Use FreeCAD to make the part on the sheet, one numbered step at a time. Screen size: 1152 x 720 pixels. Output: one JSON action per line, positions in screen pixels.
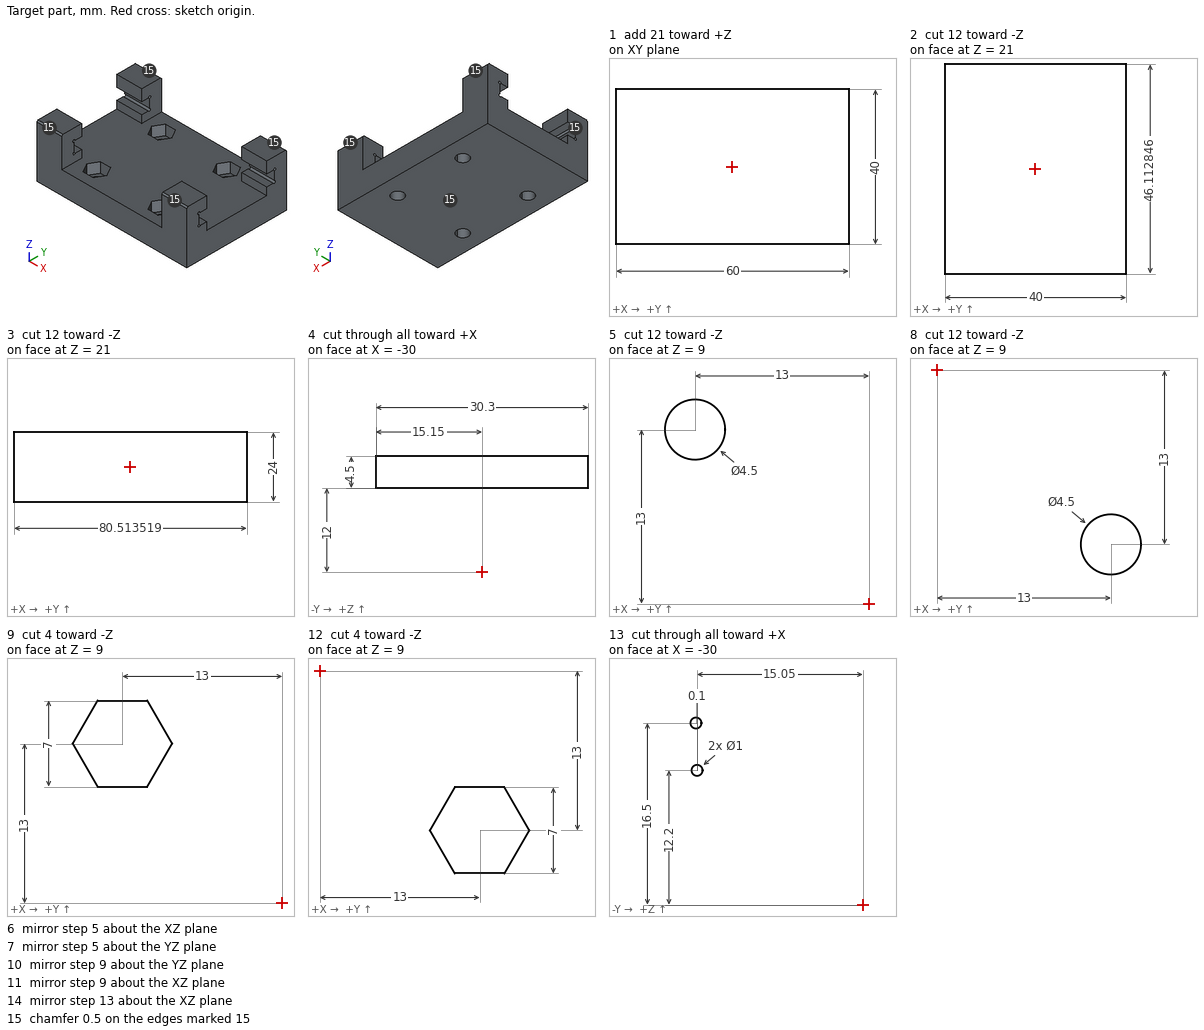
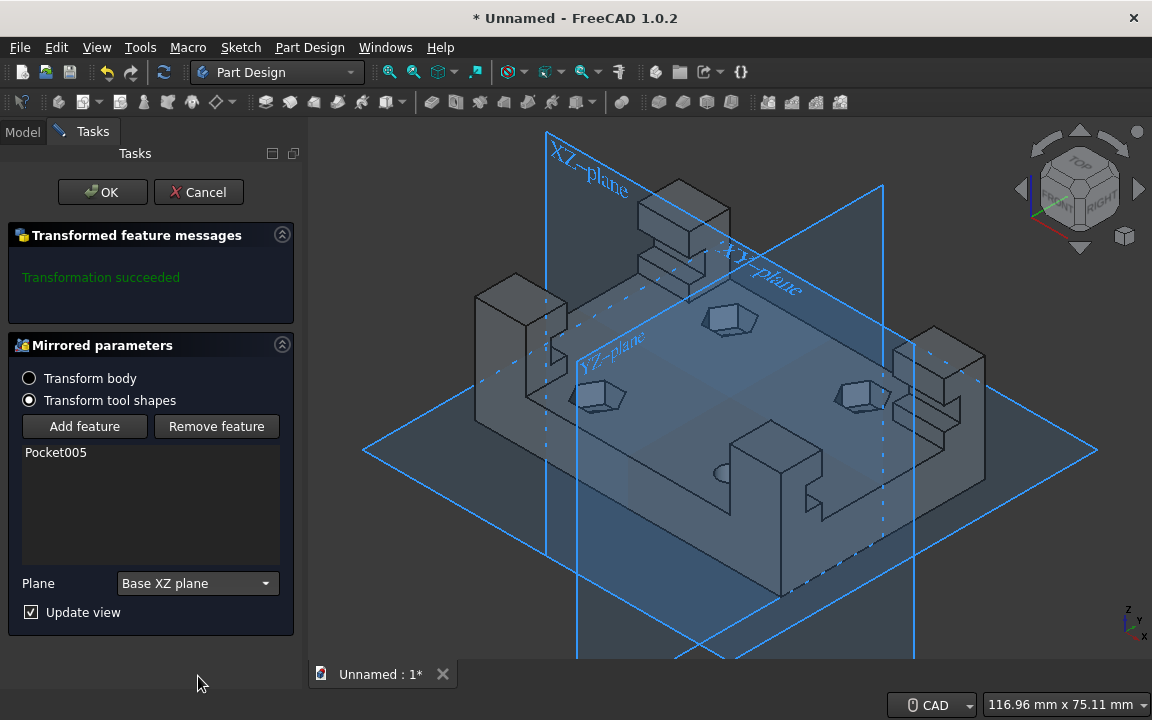
{"action": "left_click", "coordinate": [103, 192]}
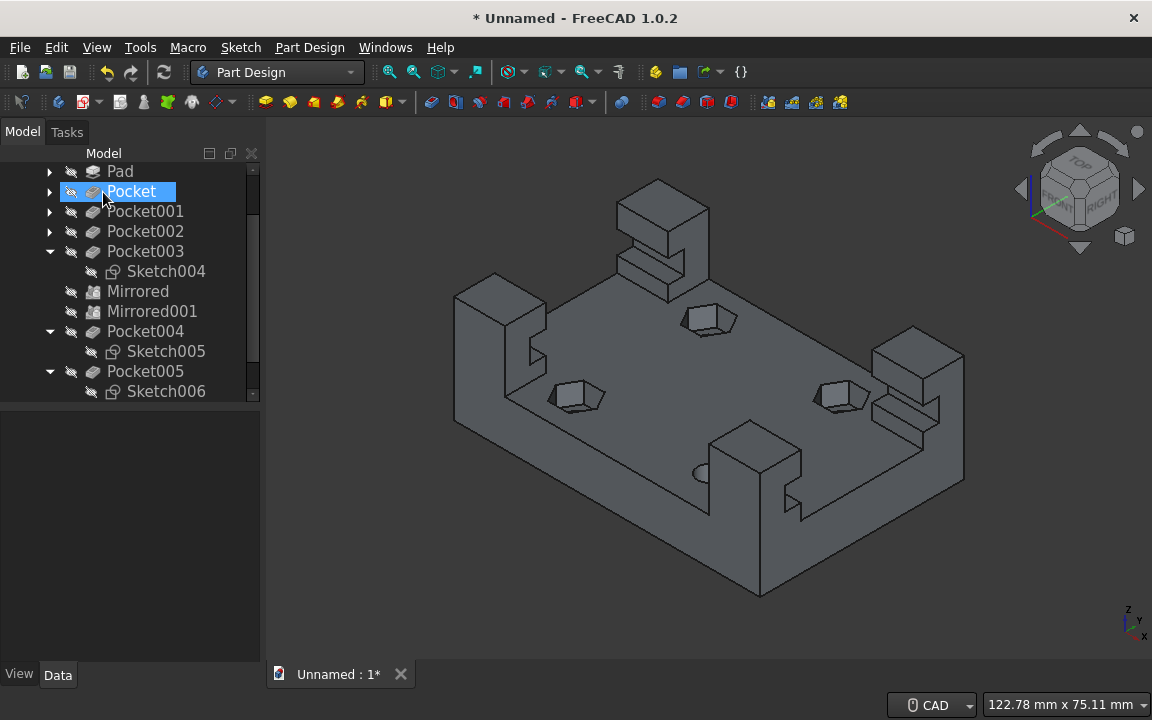
{"action": "left_click", "coordinate": [709, 396]}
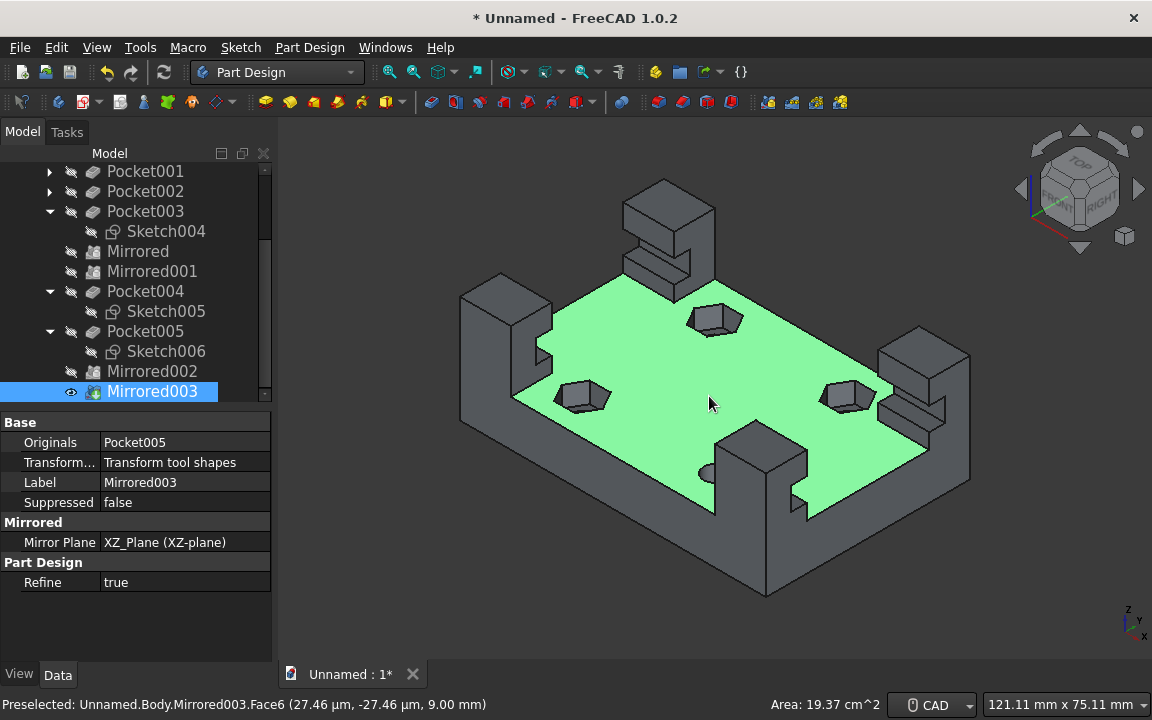
{"action": "left_click", "coordinate": [84, 102]}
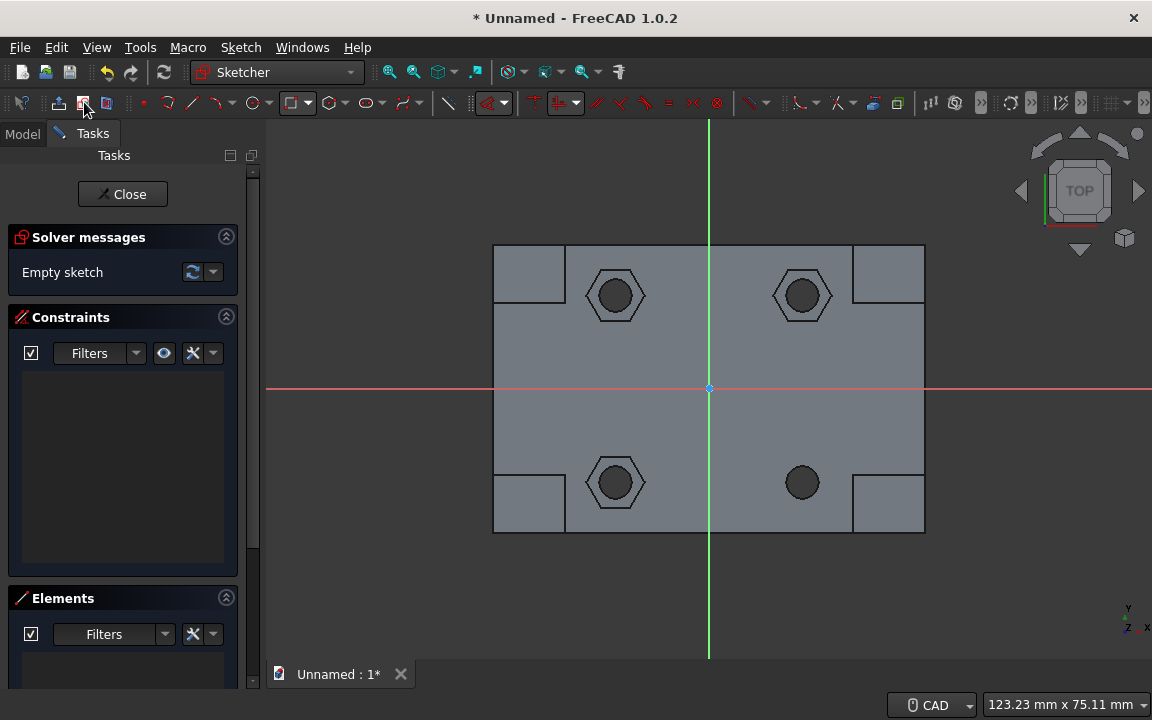
{"action": "left_click", "coordinate": [108, 104]}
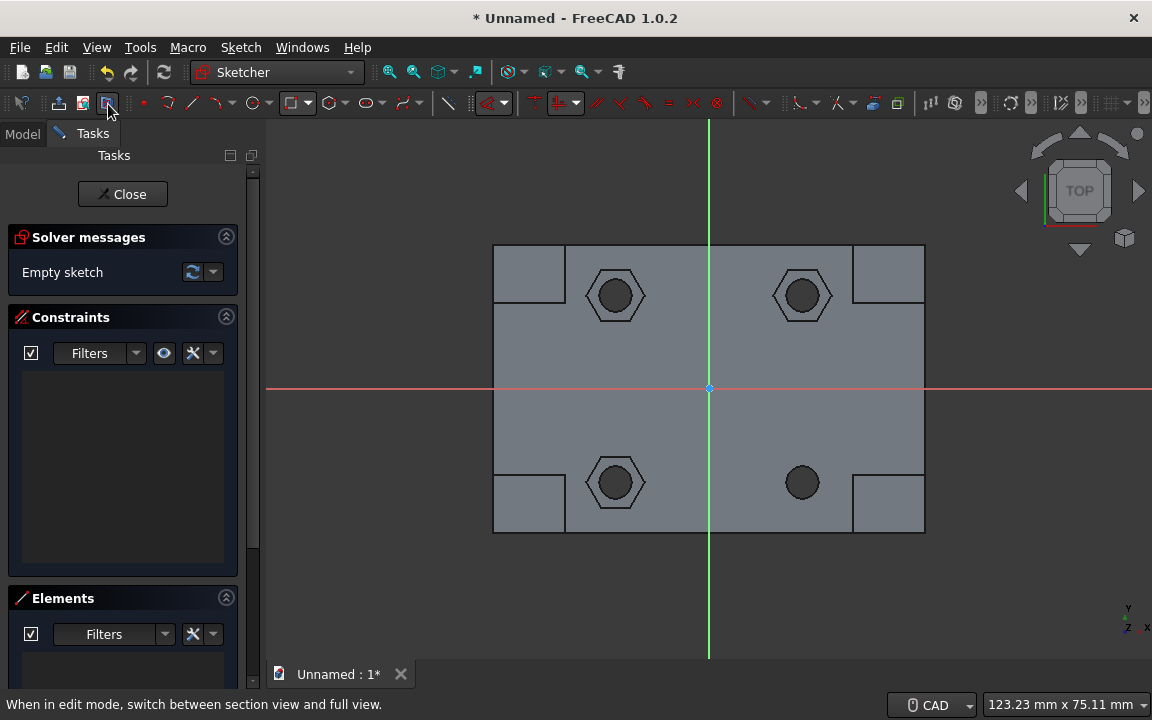
{"action": "scroll", "coordinate": [846, 483], "scroll_direction": "up", "scroll_amount": 5}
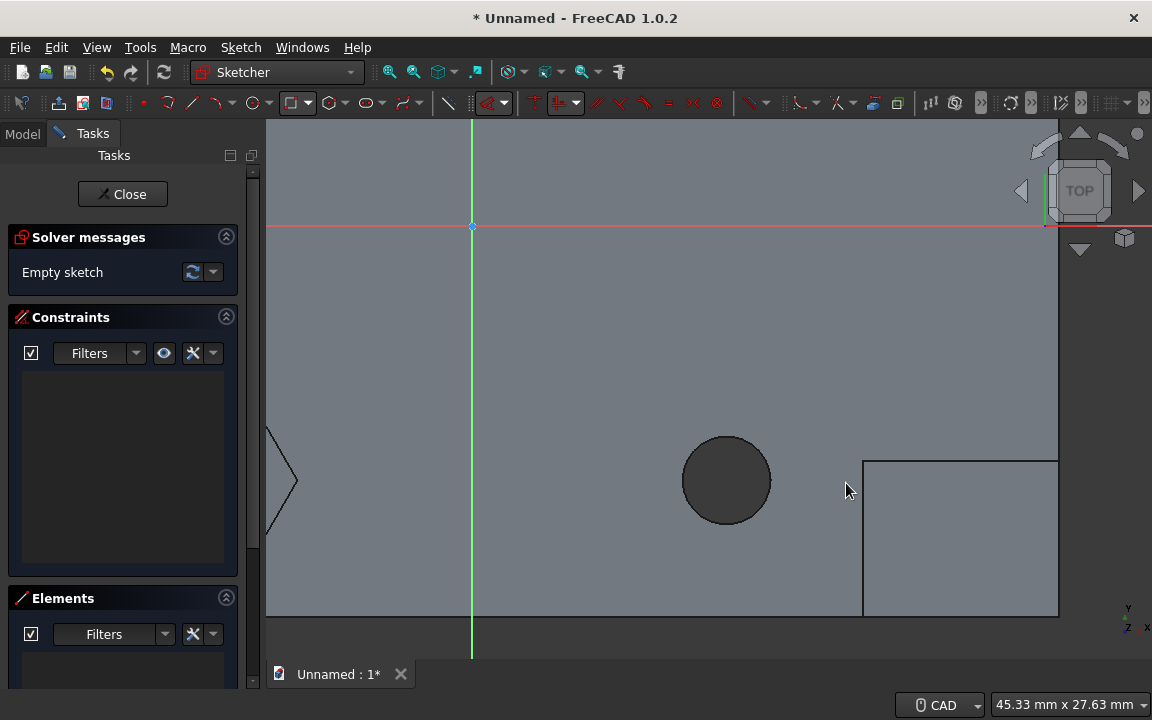
{"action": "left_click", "coordinate": [330, 104]}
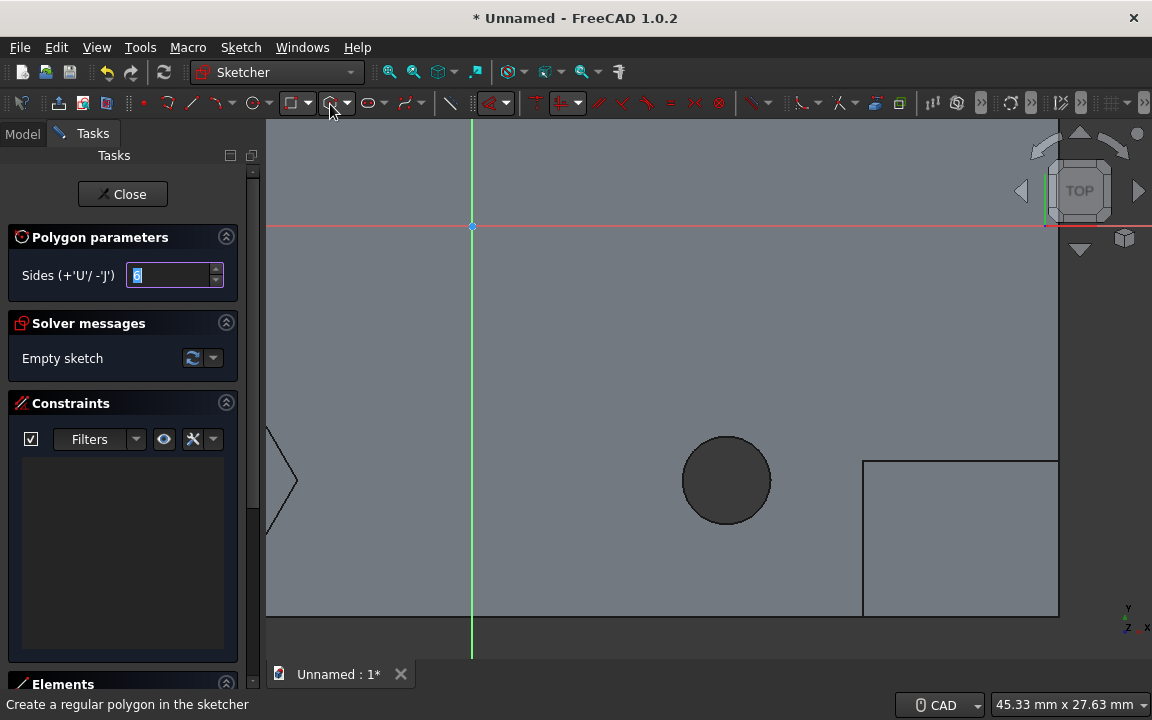
{"action": "left_click", "coordinate": [727, 480]}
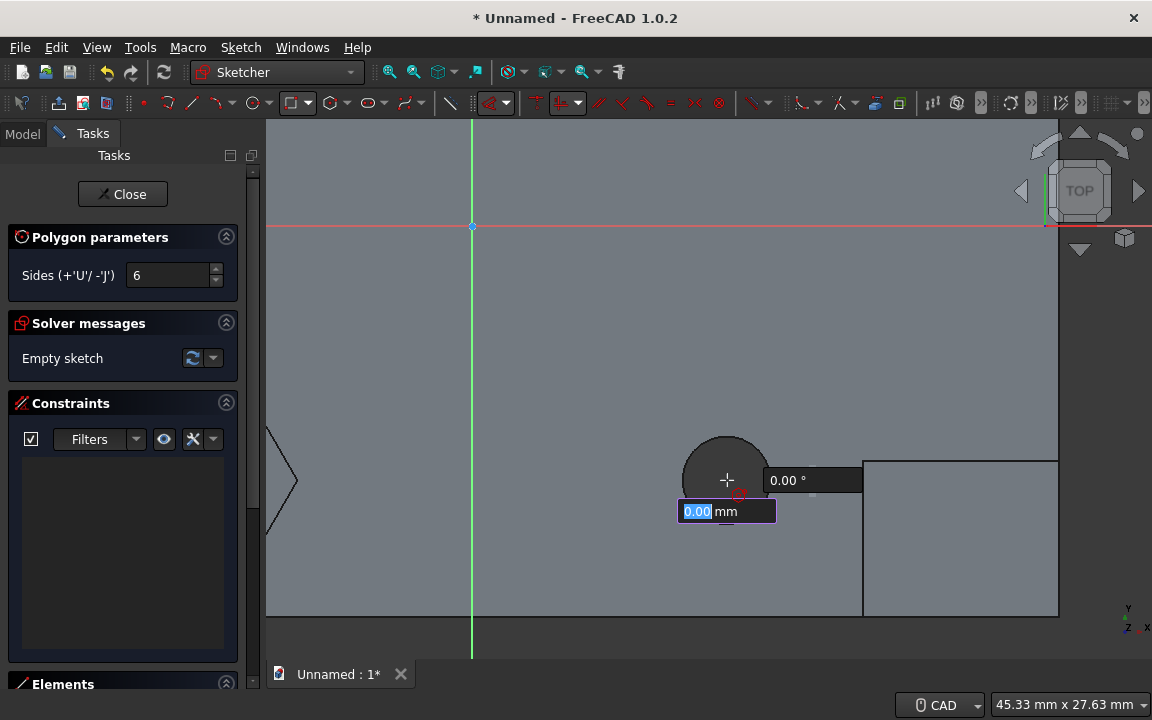
{"action": "left_click", "coordinate": [806, 480]}
{"action": "key", "text": "Escape"}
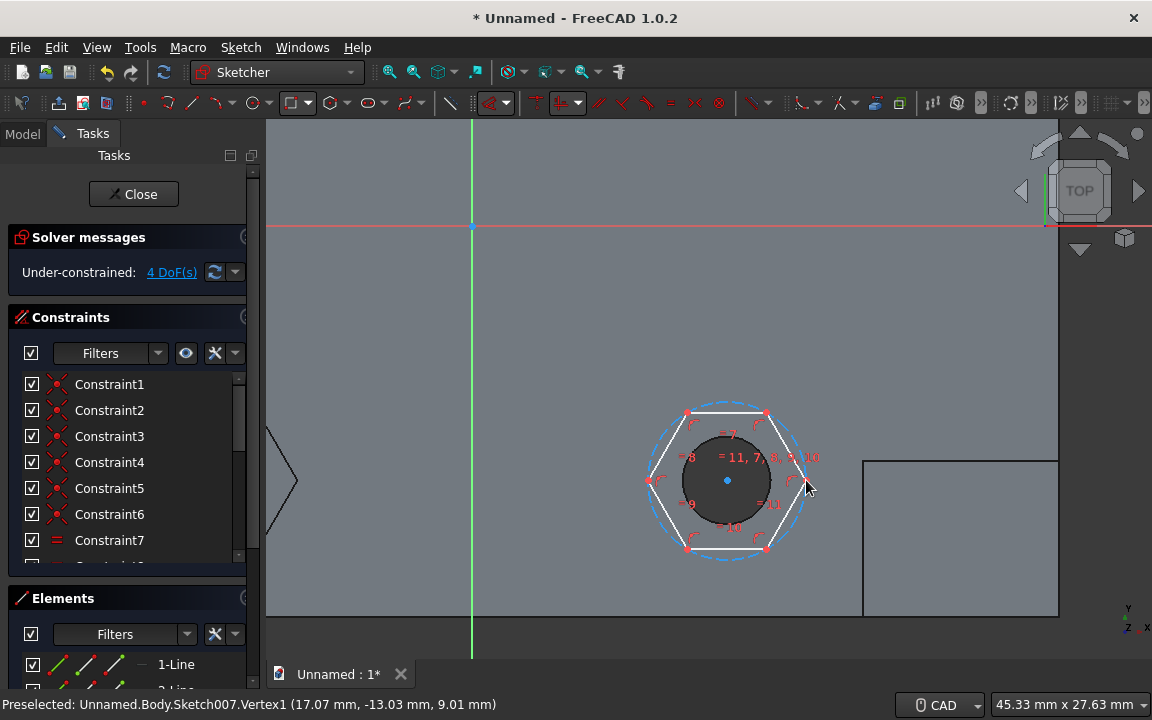
{"action": "scroll", "coordinate": [735, 413], "scroll_direction": "up", "scroll_amount": 2}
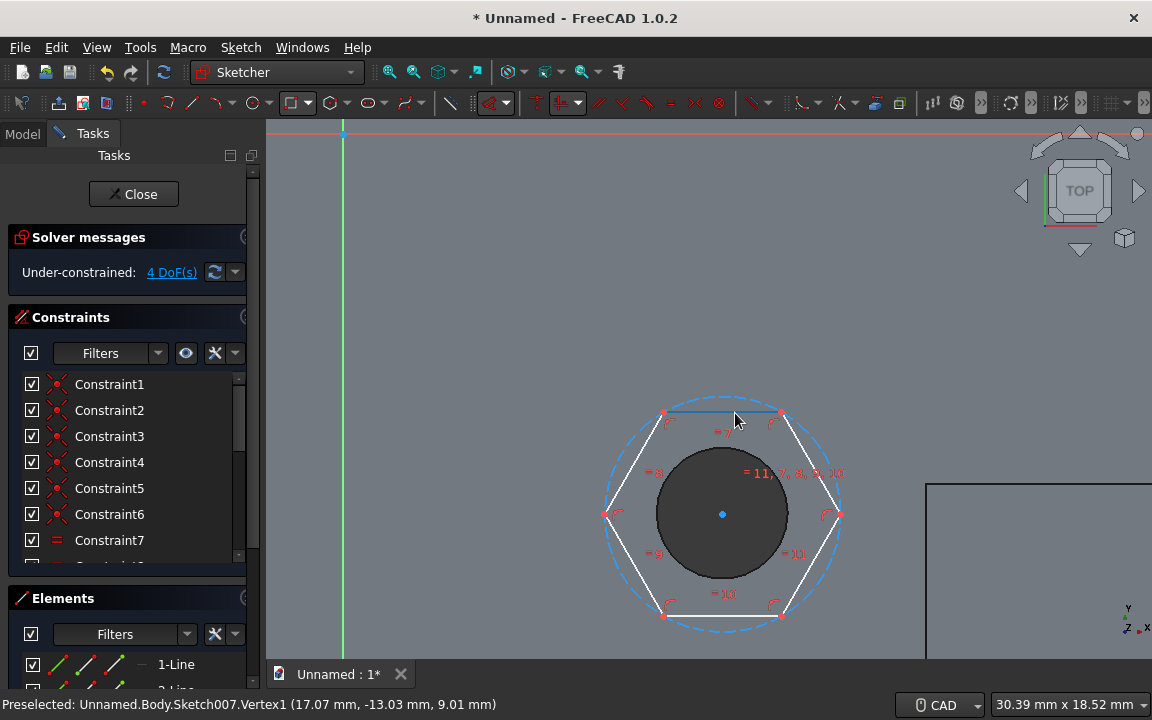
{"action": "left_click", "coordinate": [735, 412]}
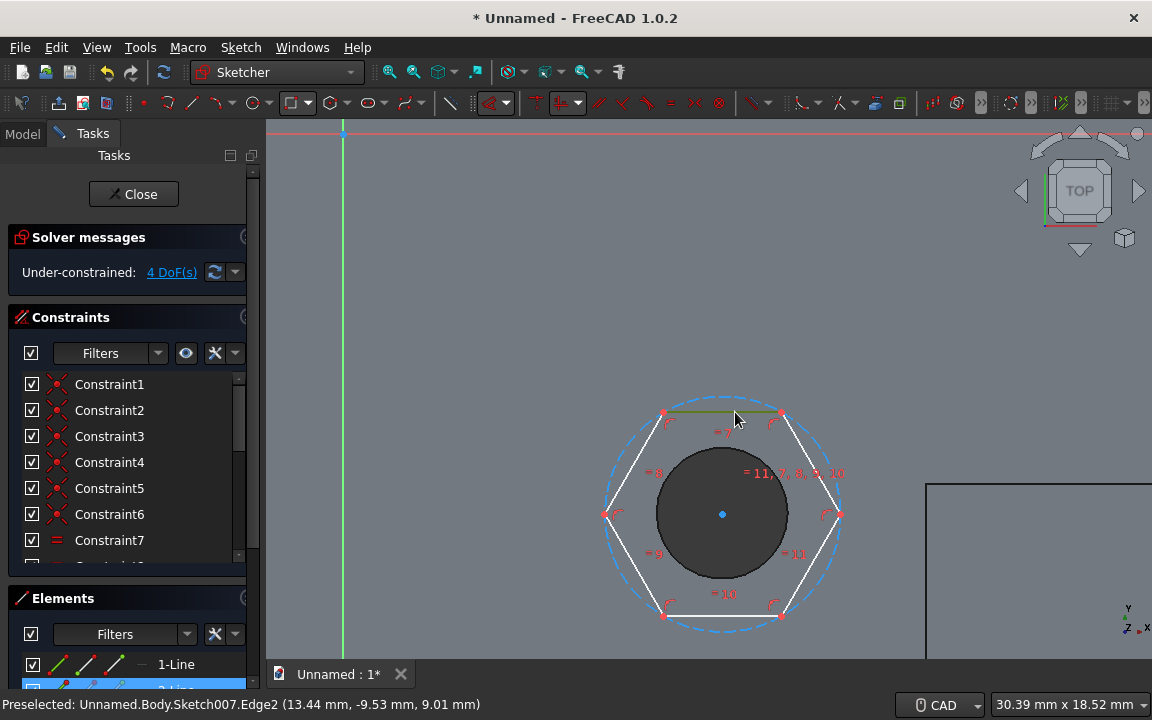
{"action": "key", "text": "h"}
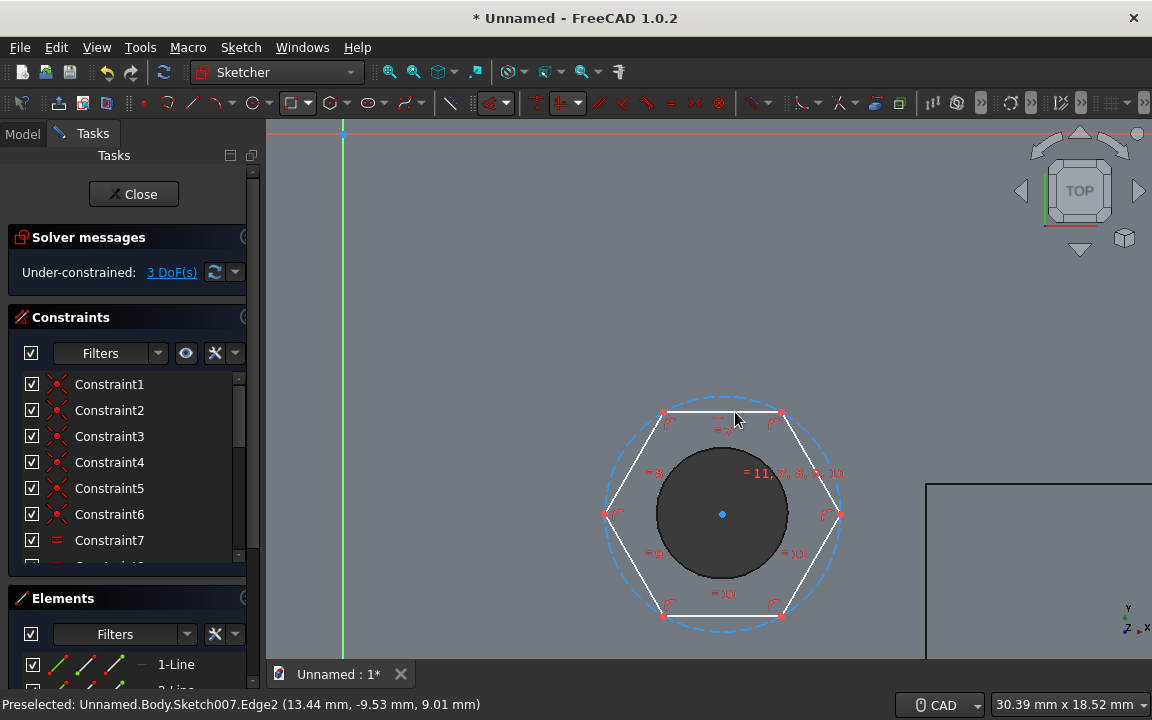
{"action": "left_click", "coordinate": [664, 616]}